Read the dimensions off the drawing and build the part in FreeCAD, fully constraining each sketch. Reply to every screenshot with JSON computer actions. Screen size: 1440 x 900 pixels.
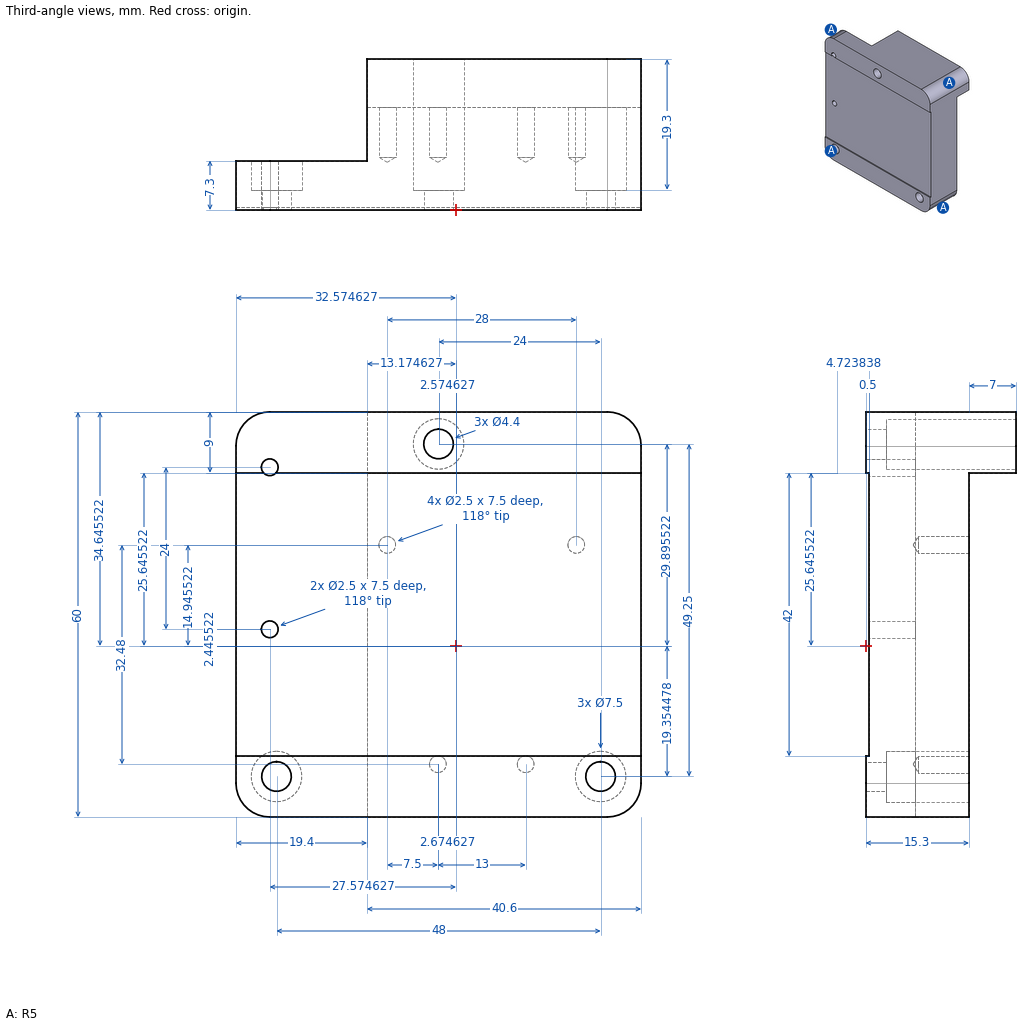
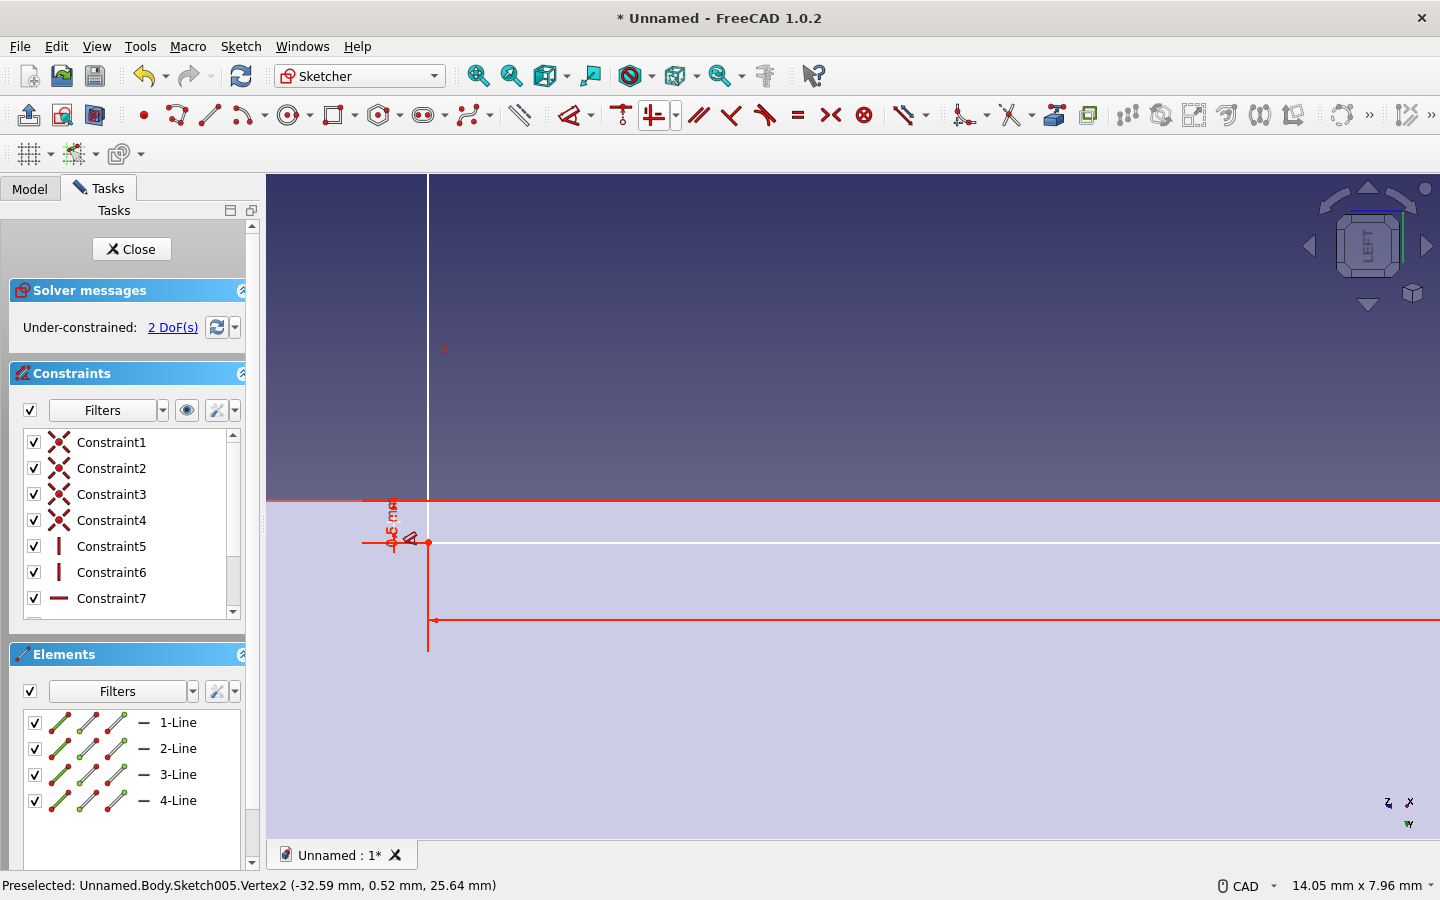
{"action": "scroll", "coordinate": [431, 547], "scroll_direction": "down", "scroll_amount": 8}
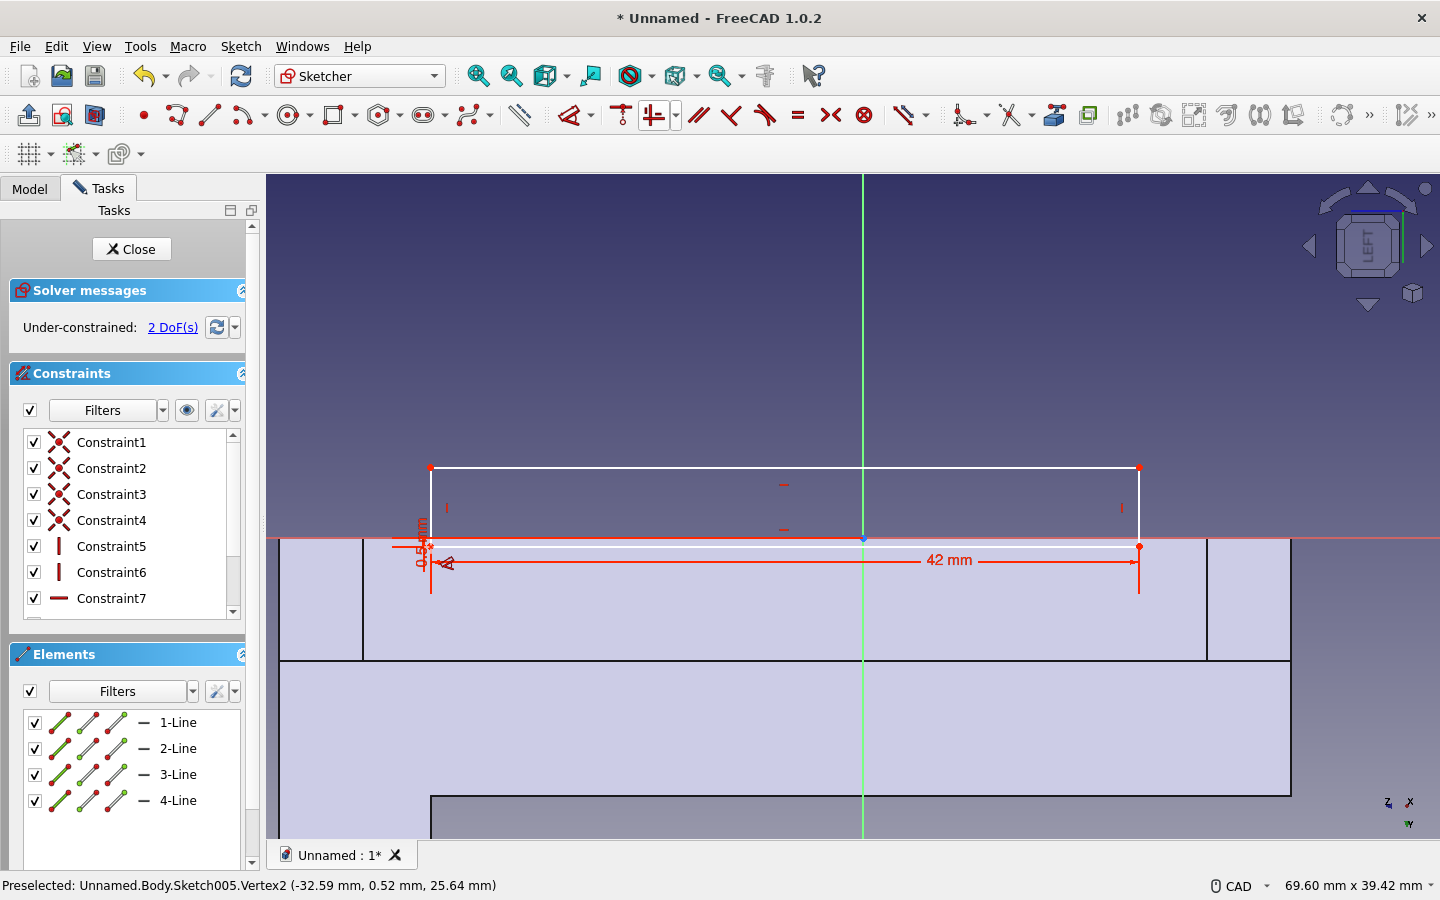
{"action": "left_click", "coordinate": [431, 492]}
{"action": "left_click", "coordinate": [397, 507]}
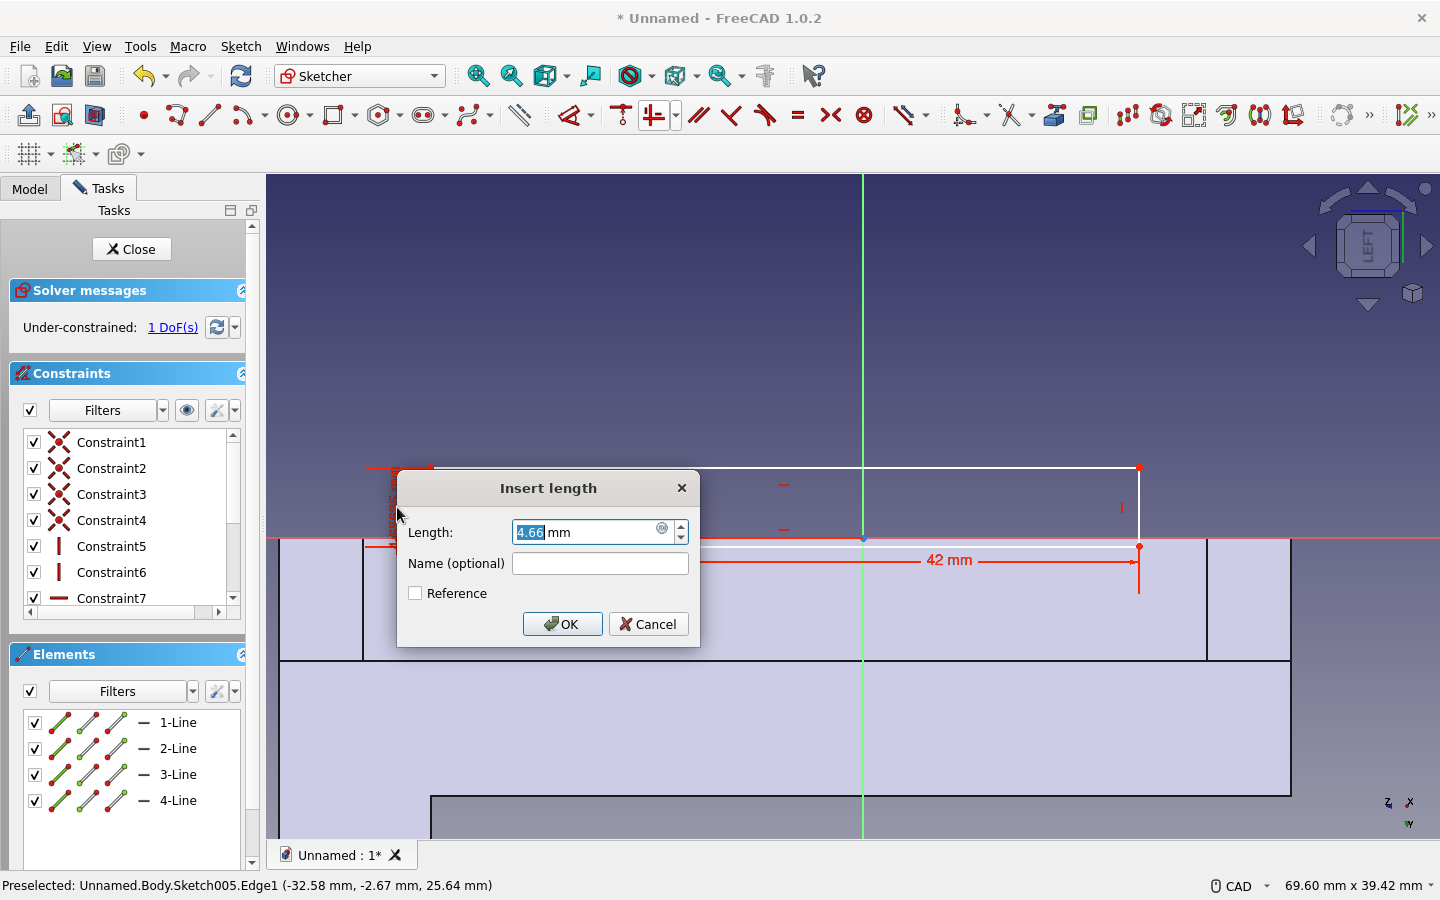
{"action": "type", "text": "4.723838"}
{"action": "key", "text": "Return"}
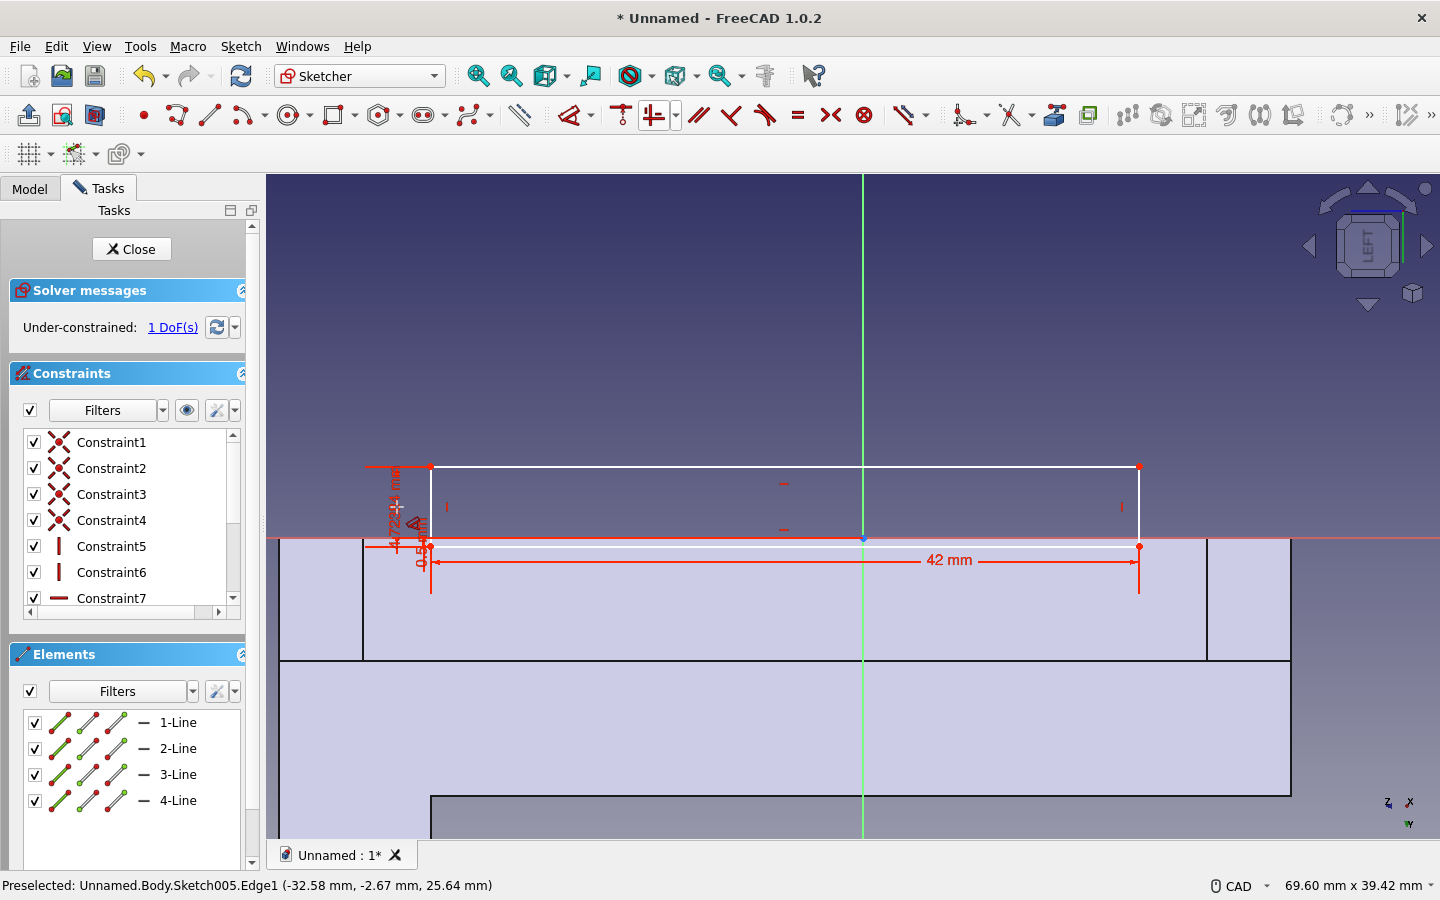
{"action": "left_click", "coordinate": [431, 467]}
{"action": "left_click", "coordinate": [647, 433]}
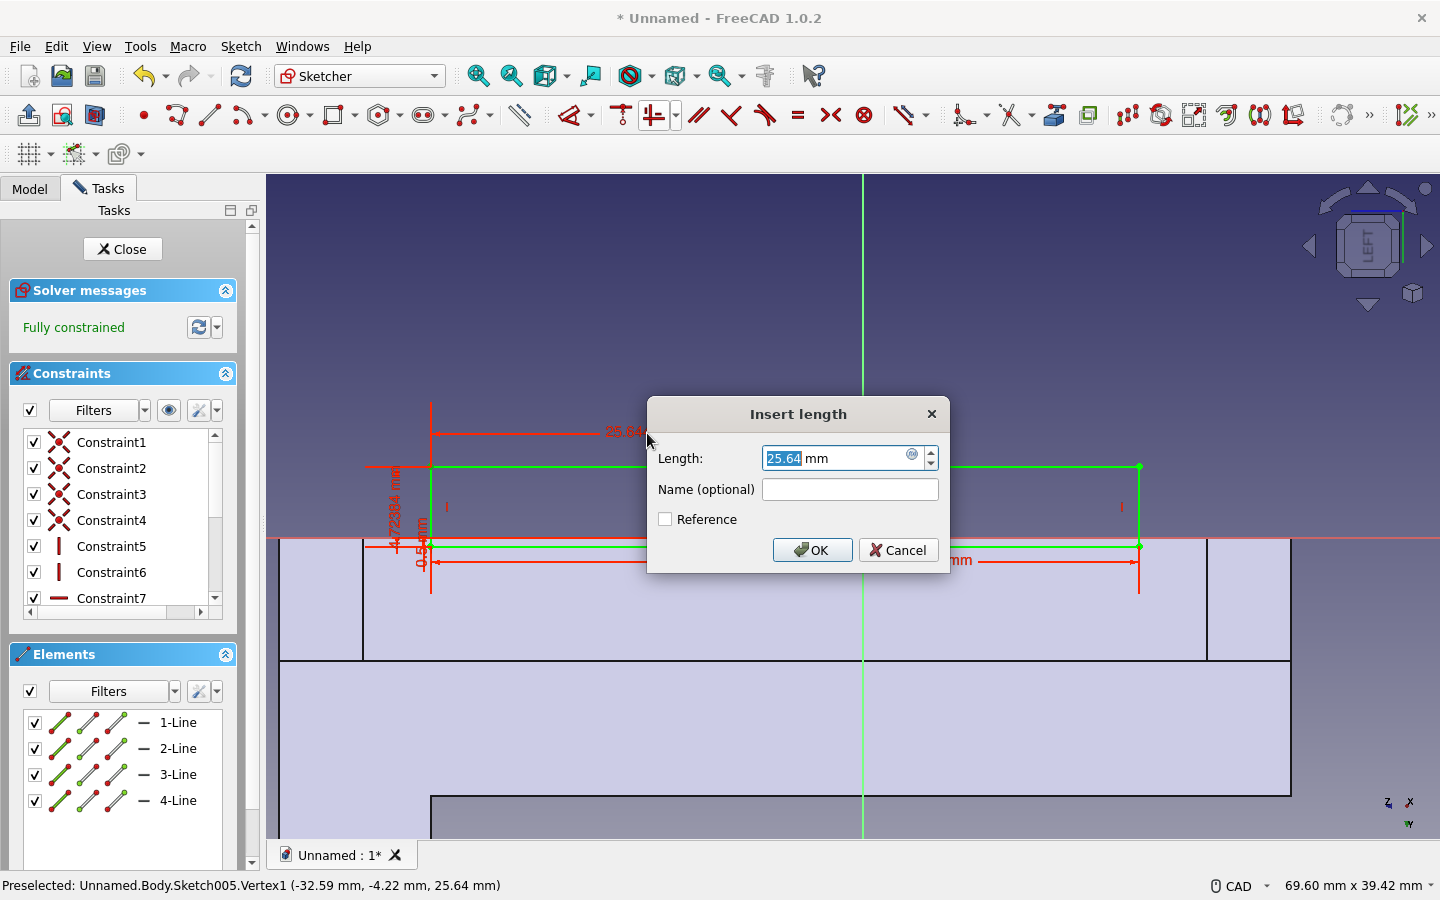
{"action": "type", "text": "25.645522"}
{"action": "key", "text": "Return"}
{"action": "key", "text": "Escape"}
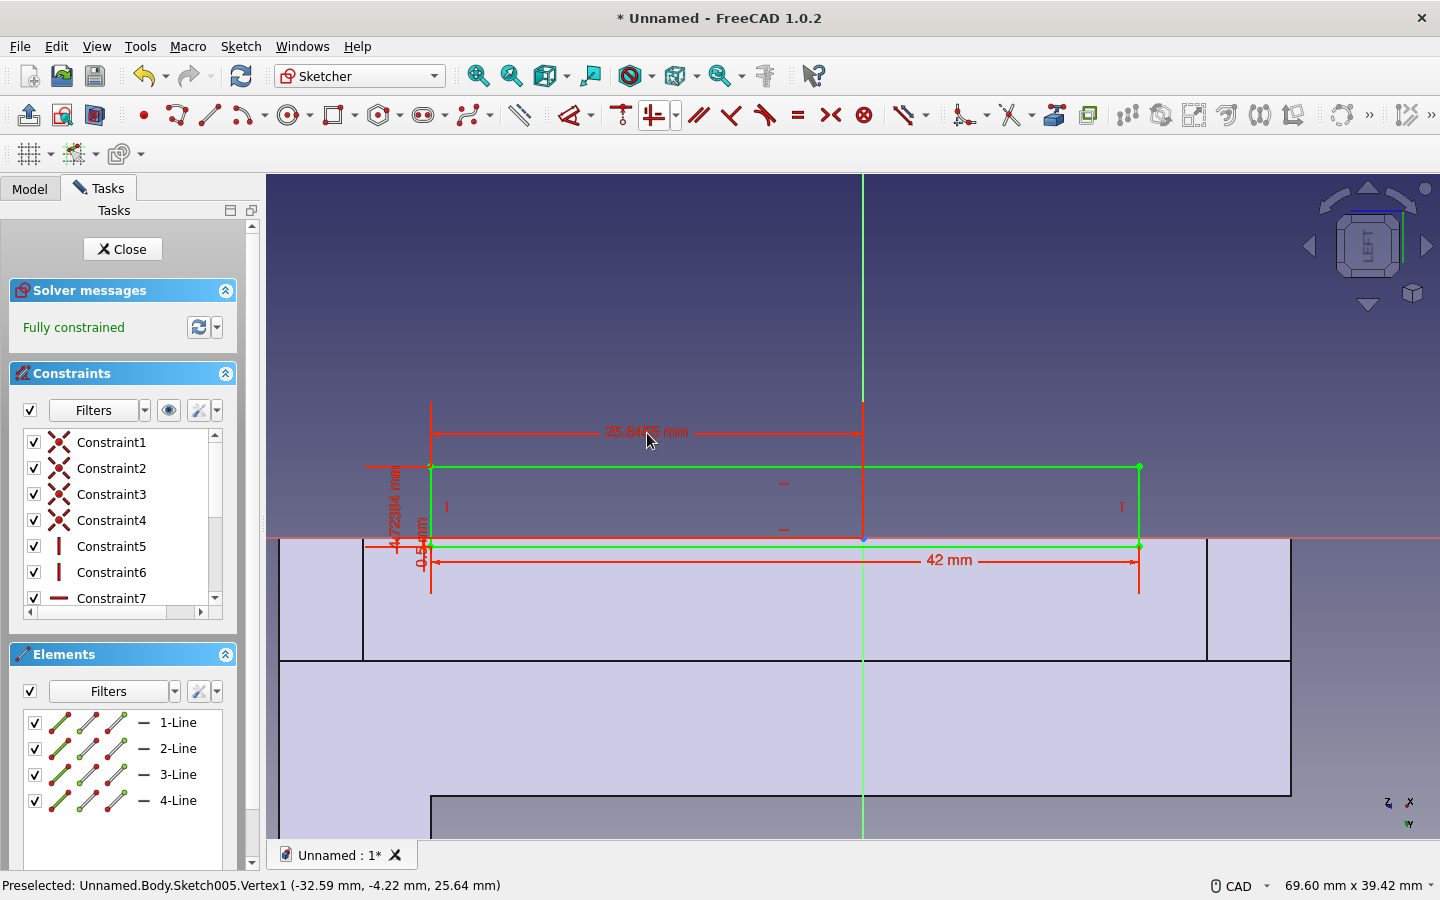
{"action": "left_click", "coordinate": [123, 249]}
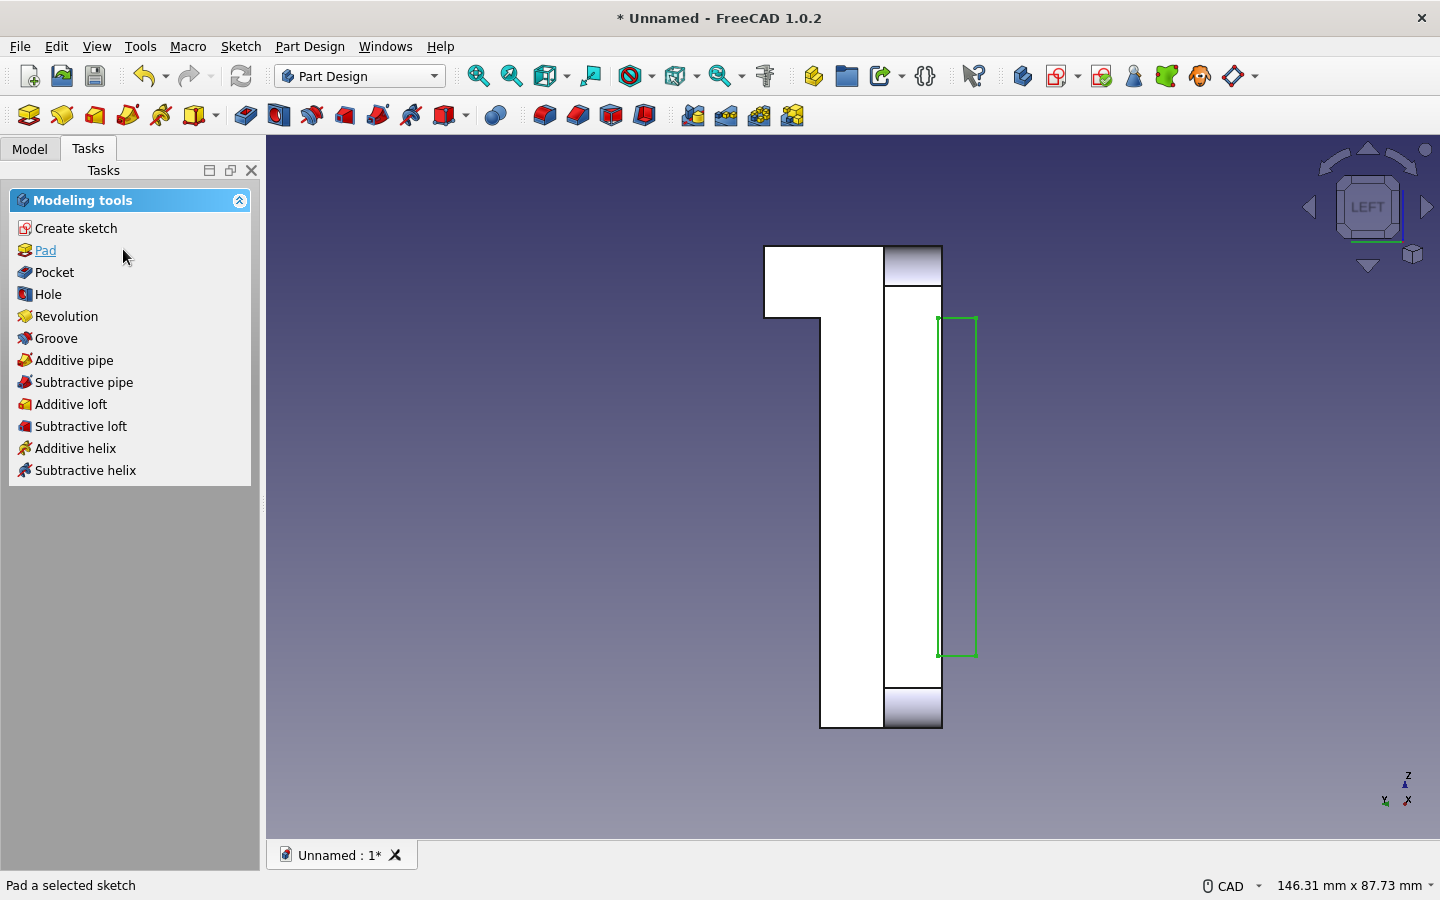
{"action": "left_click", "coordinate": [246, 116]}